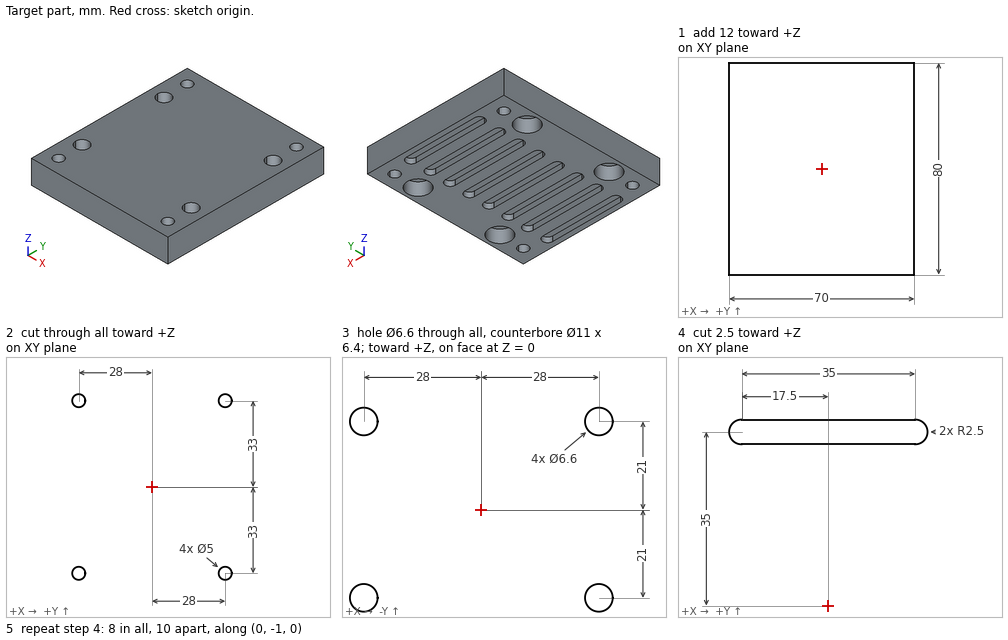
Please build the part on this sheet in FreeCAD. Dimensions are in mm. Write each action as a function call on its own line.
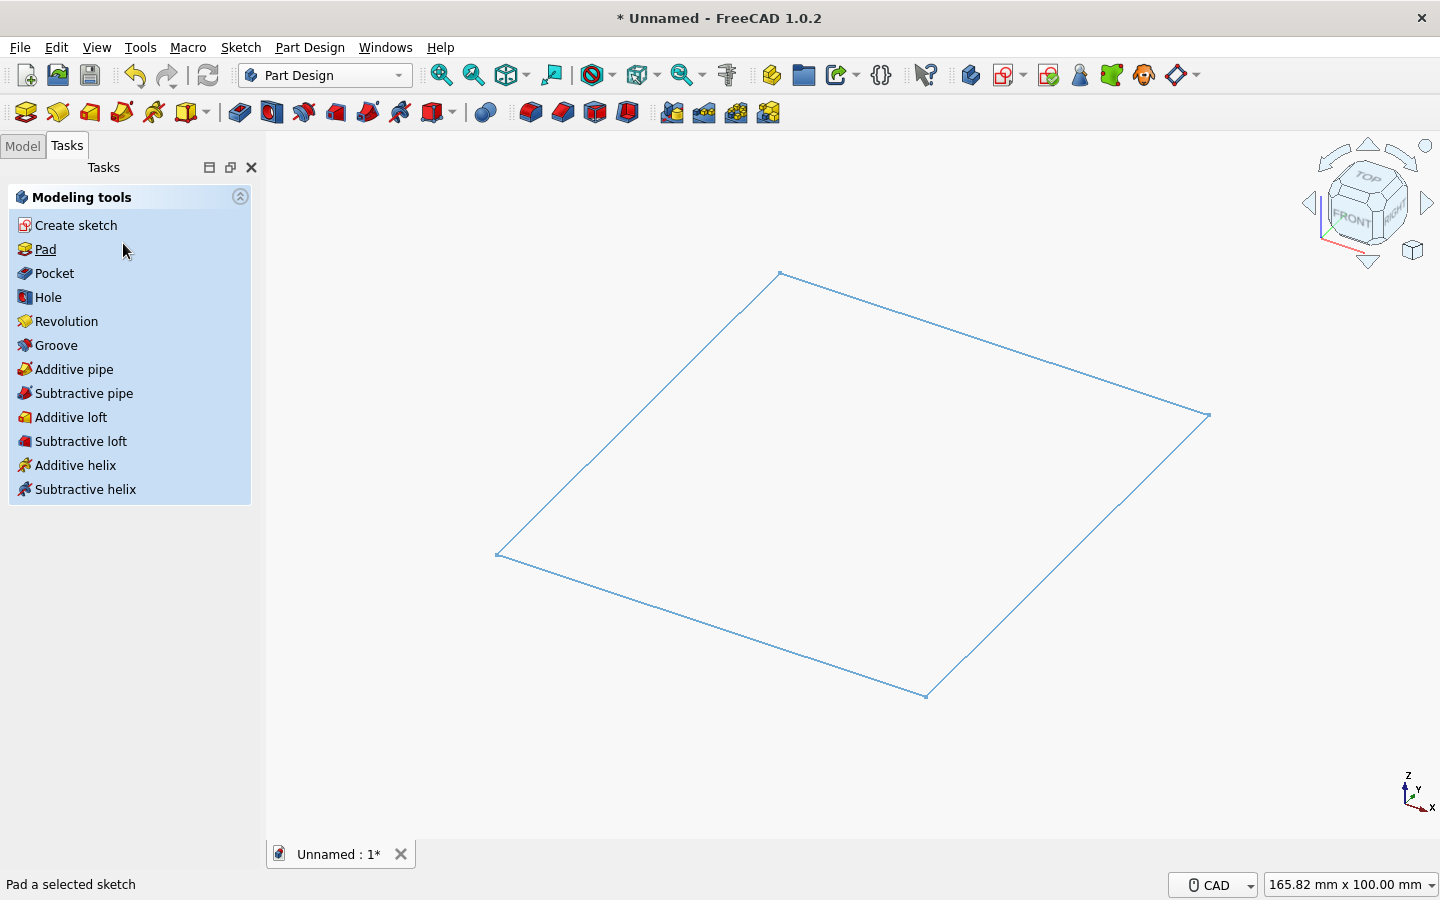
click(26, 112)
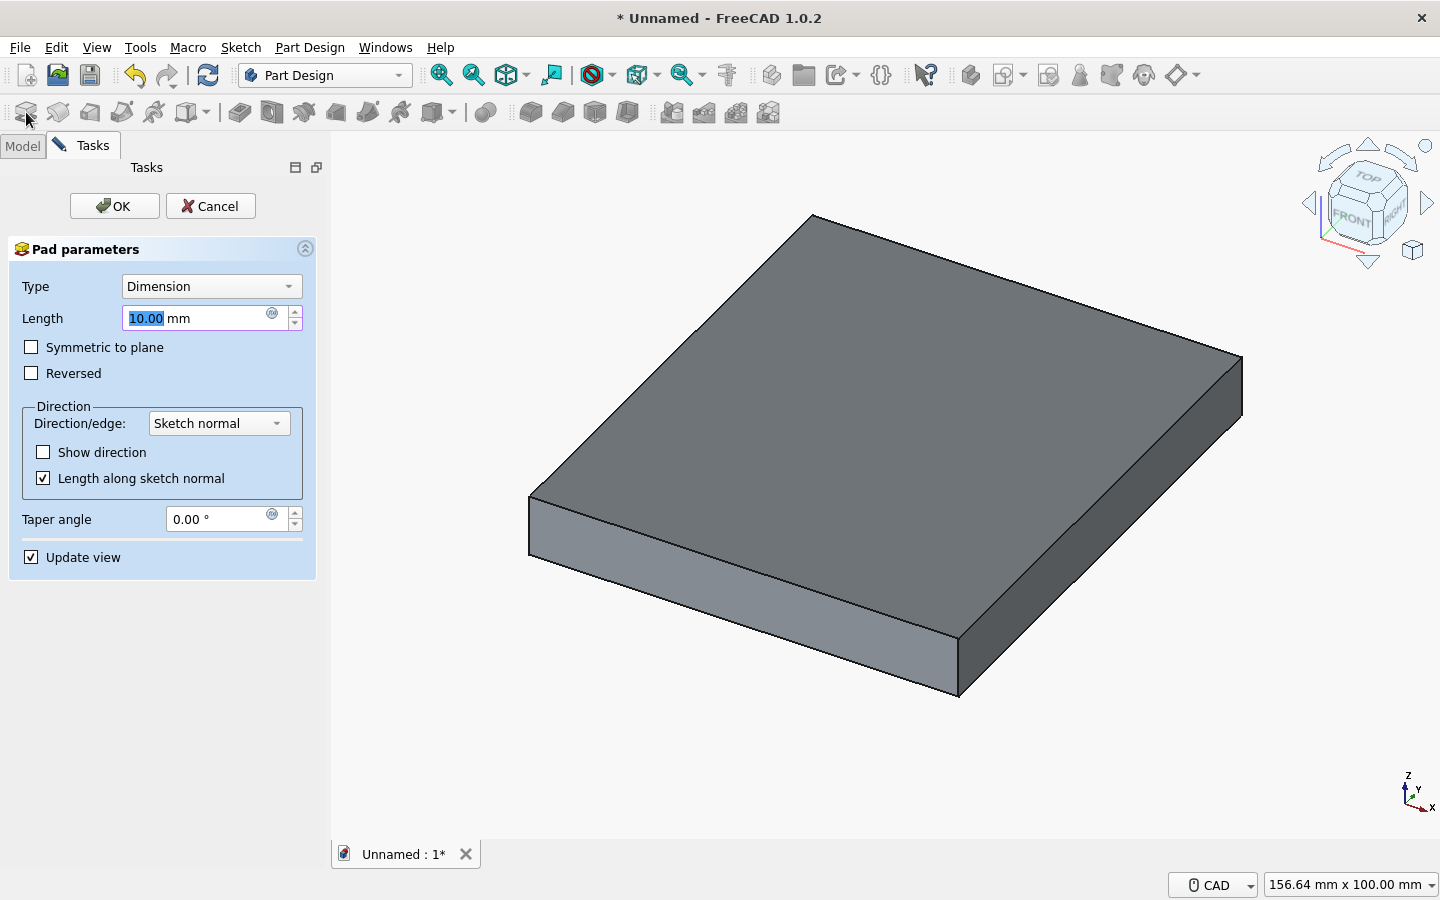
text(12)
key(Tab)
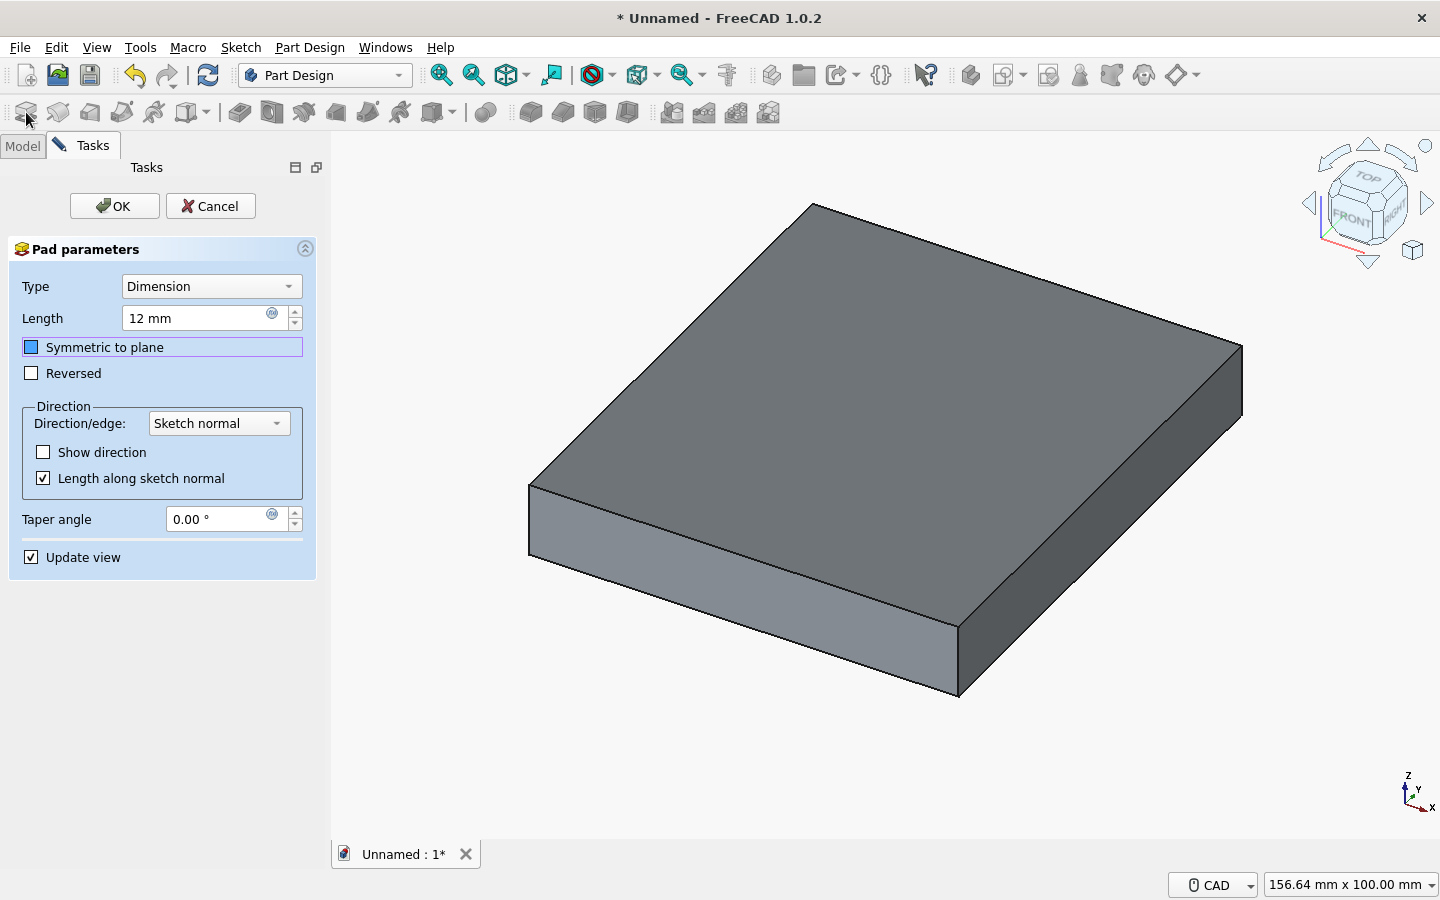
click(115, 206)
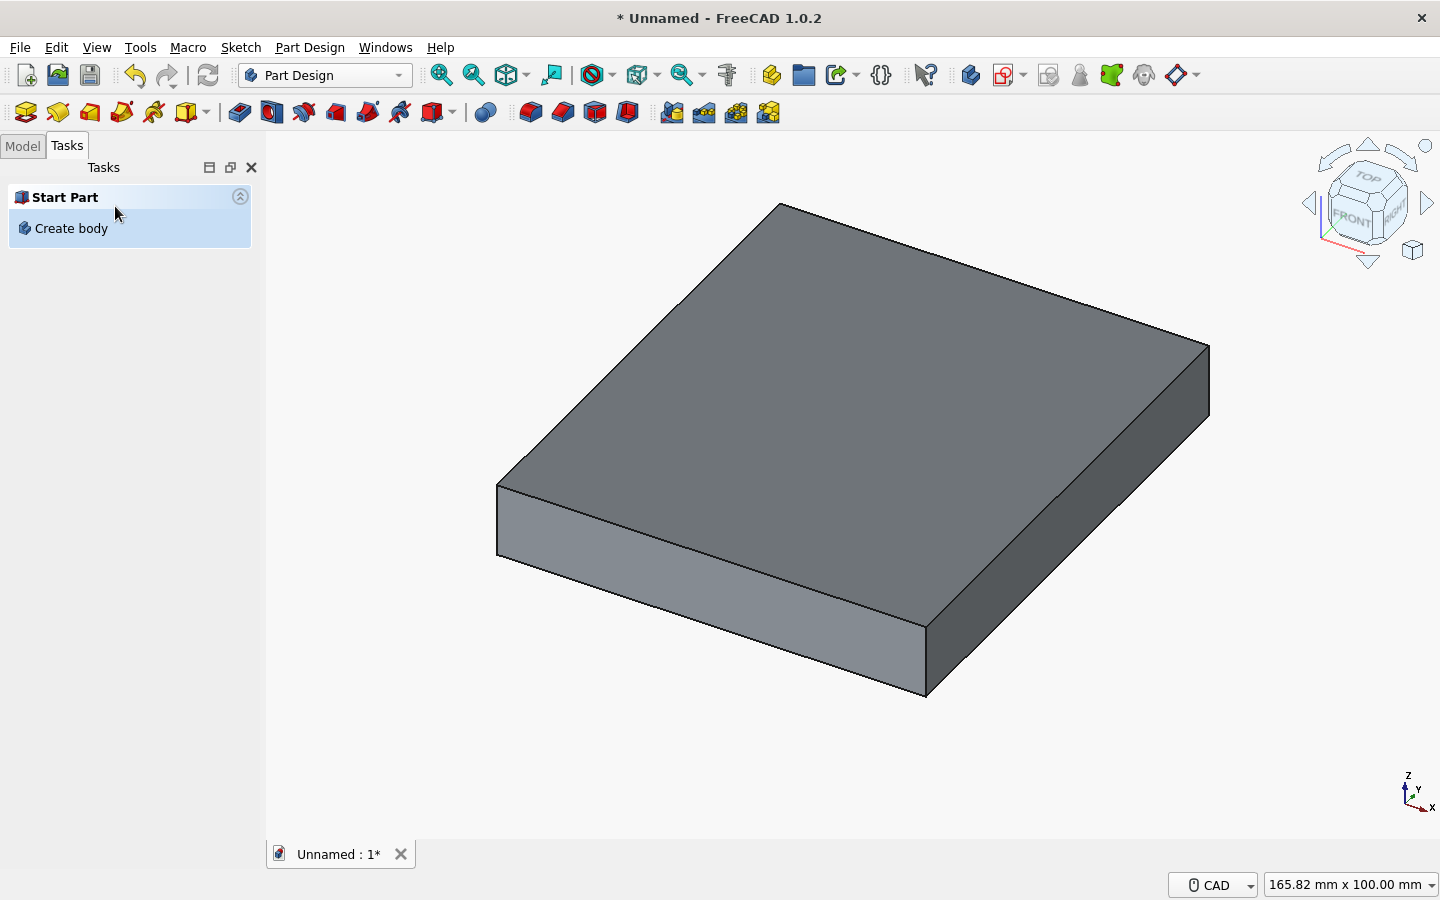
click(1004, 76)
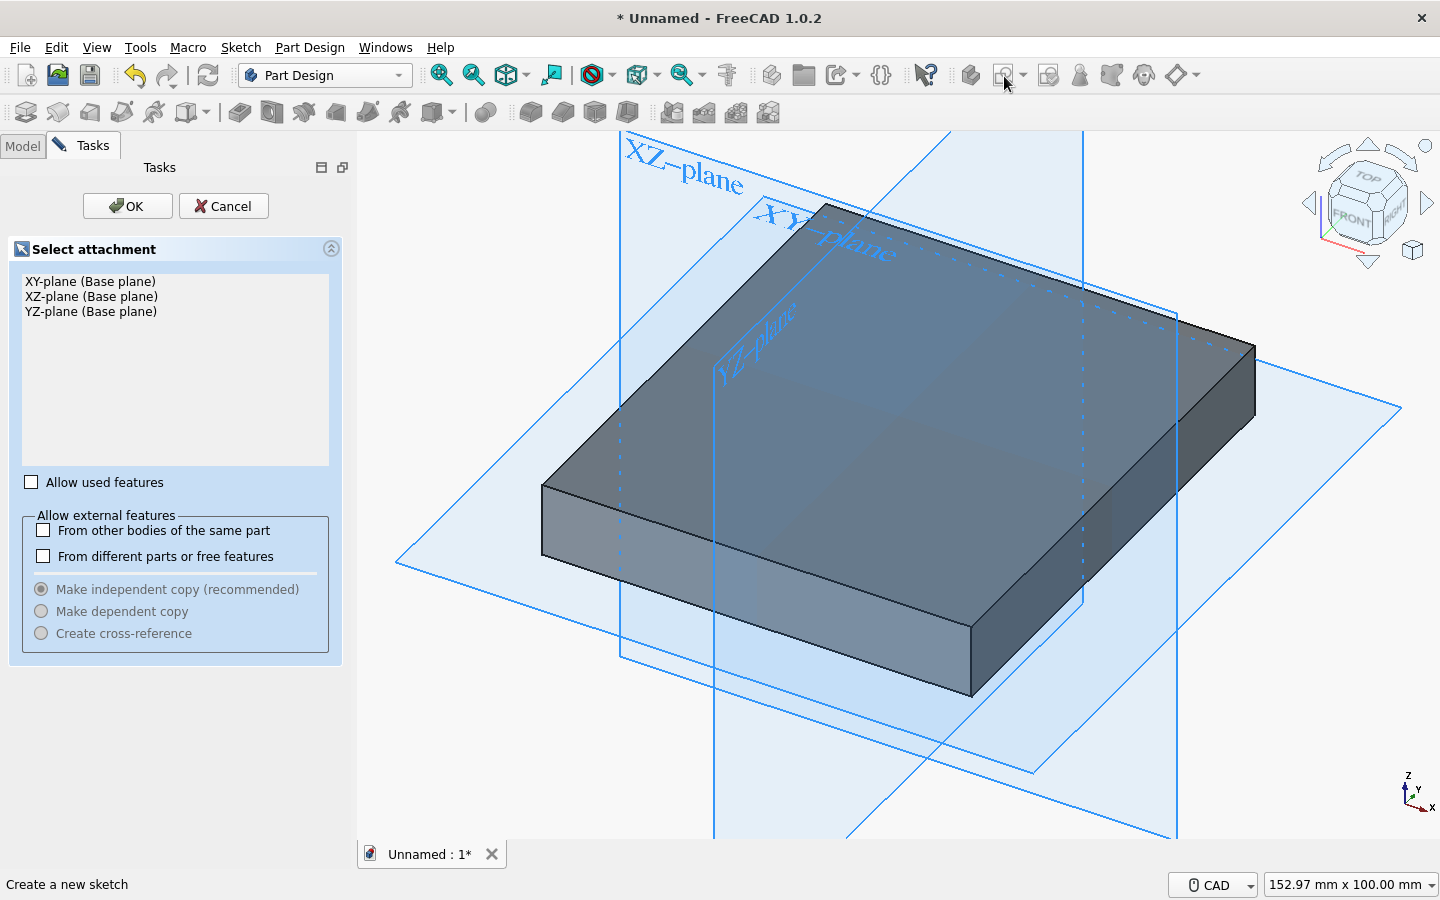
click(82, 282)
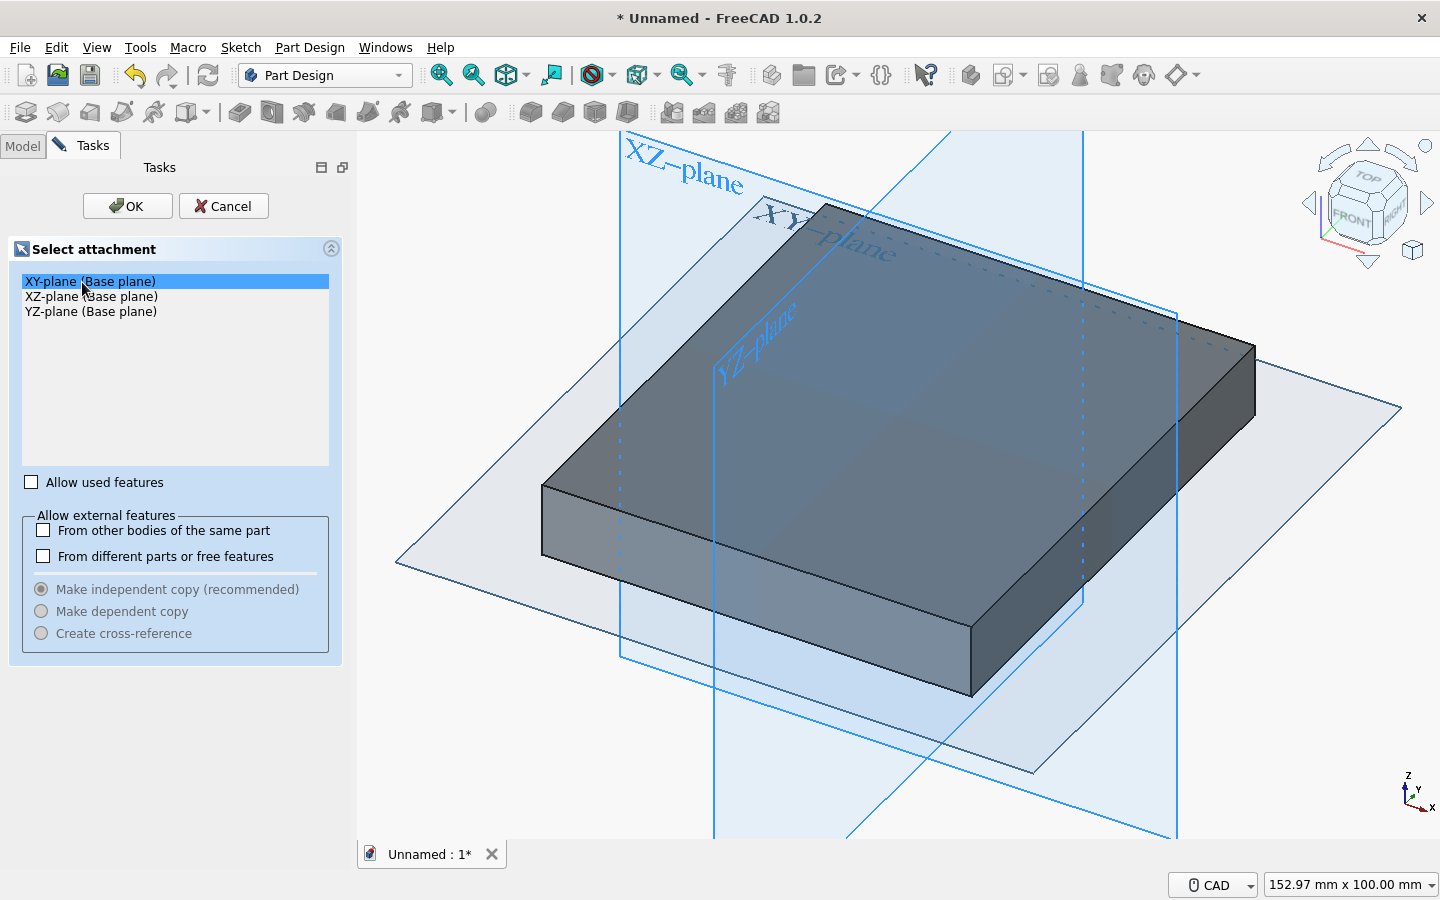
click(128, 206)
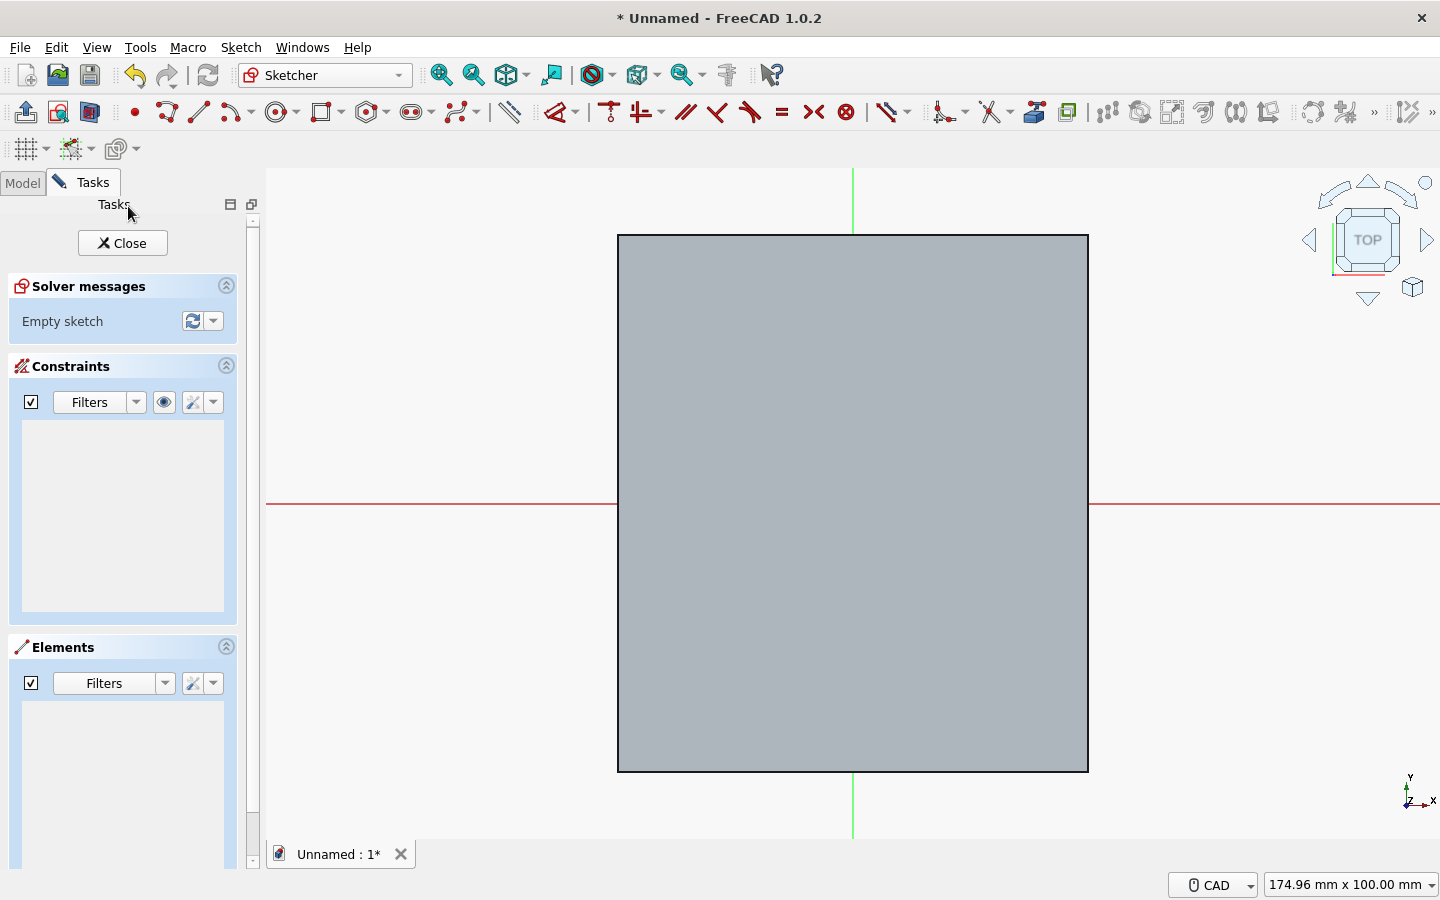
click(90, 112)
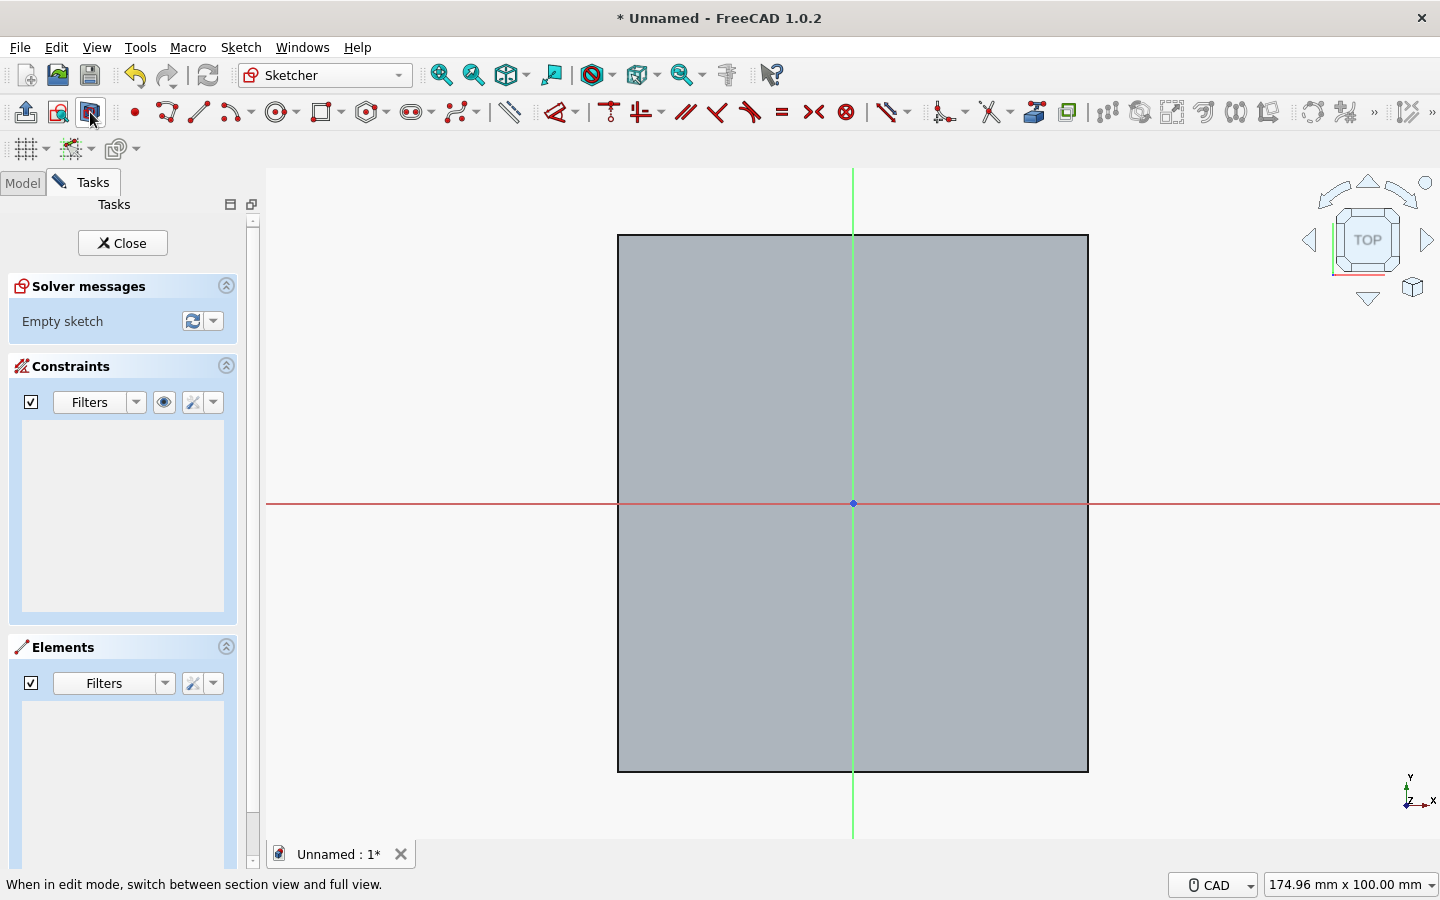
click(276, 112)